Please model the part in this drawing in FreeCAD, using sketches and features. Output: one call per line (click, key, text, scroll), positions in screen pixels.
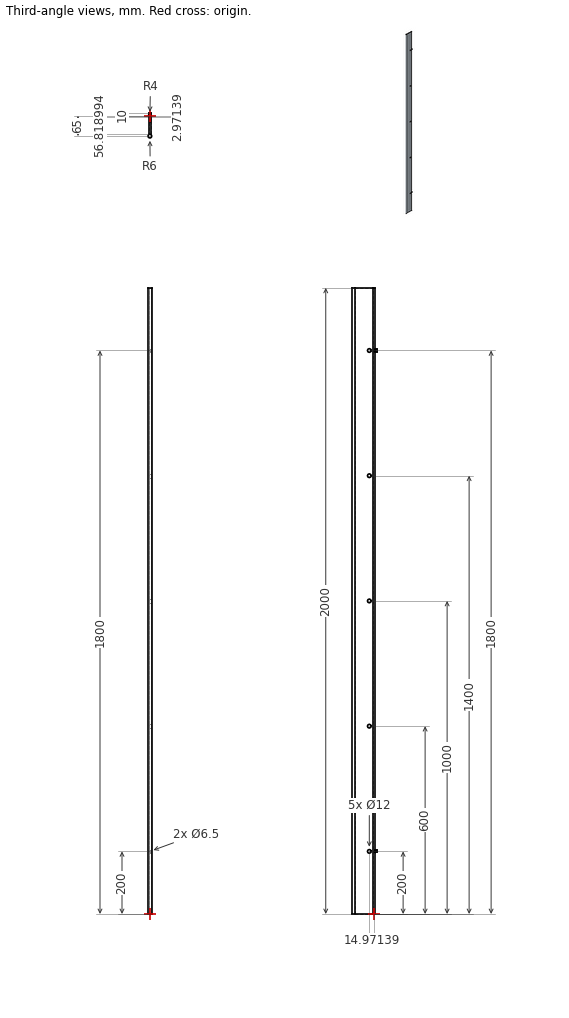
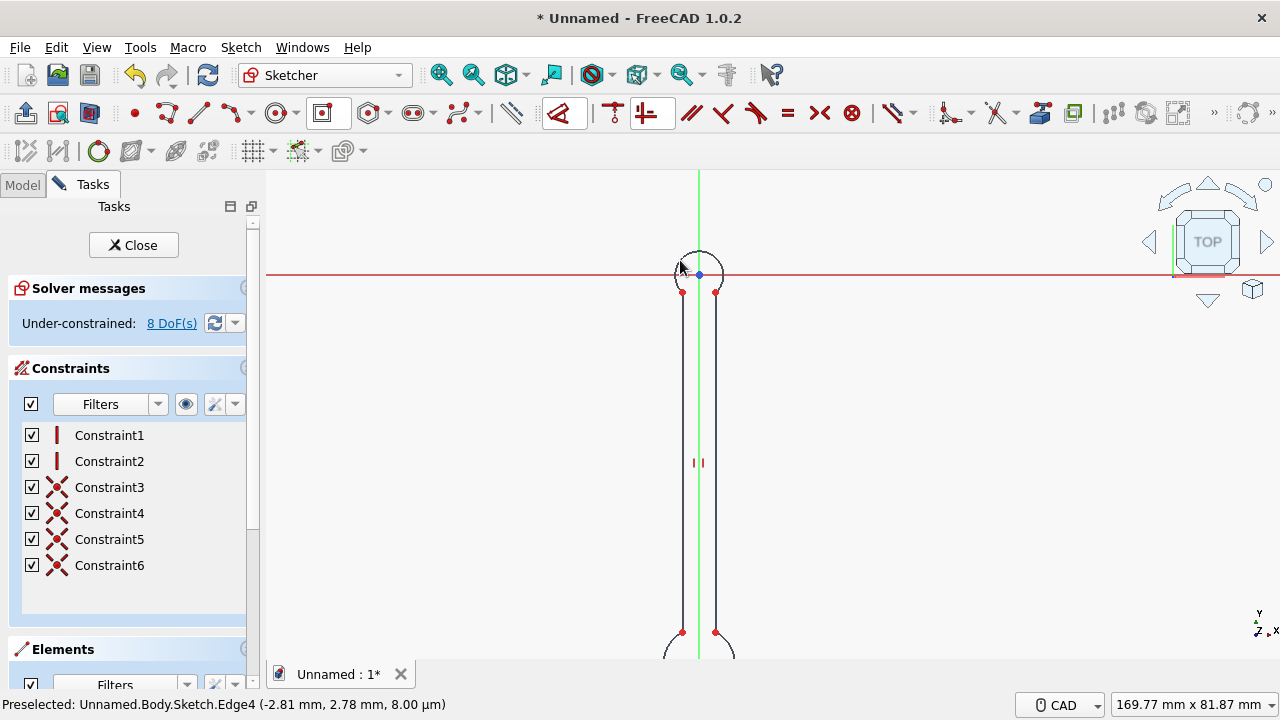
scroll(699, 275, up, 3)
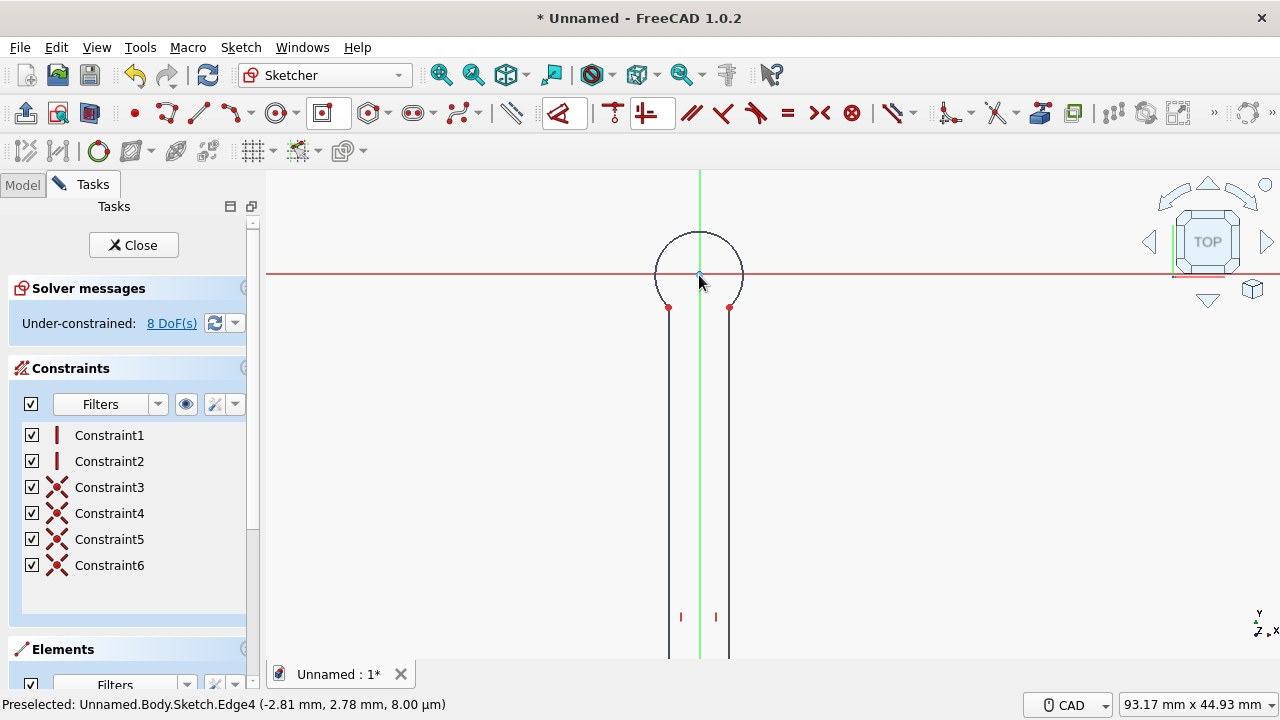
drag(689, 264, 710, 286)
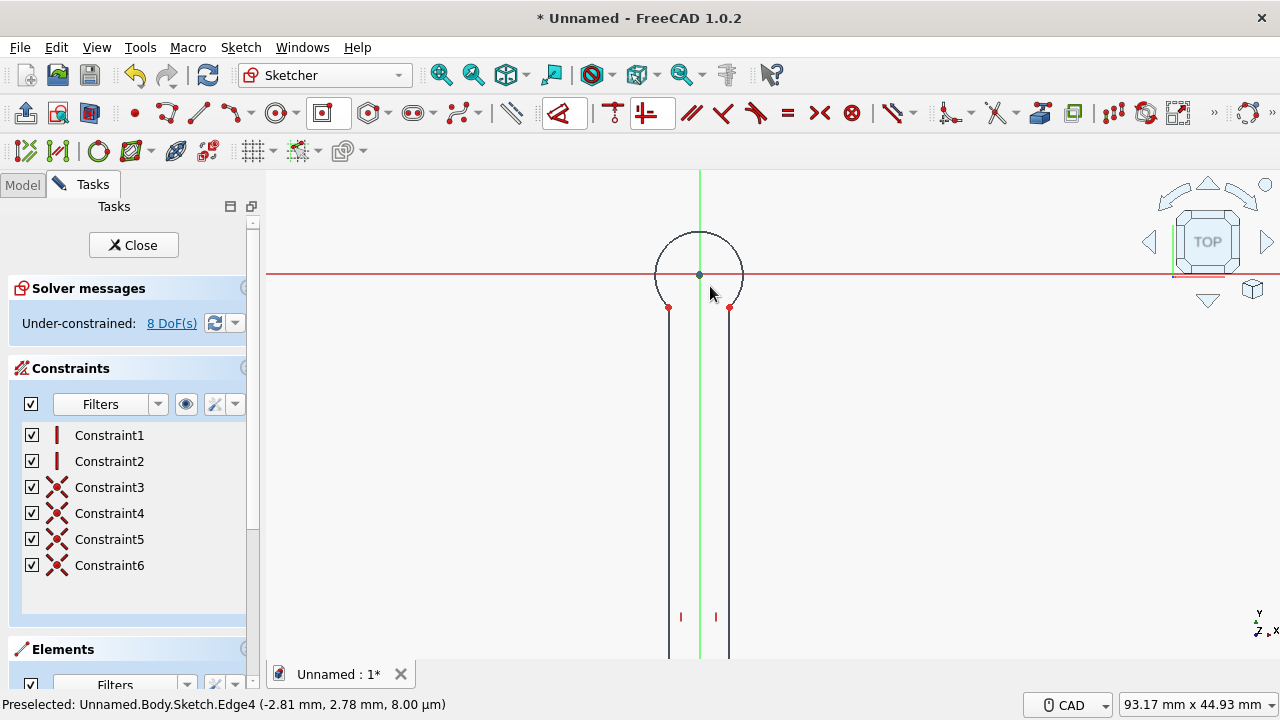
key(c)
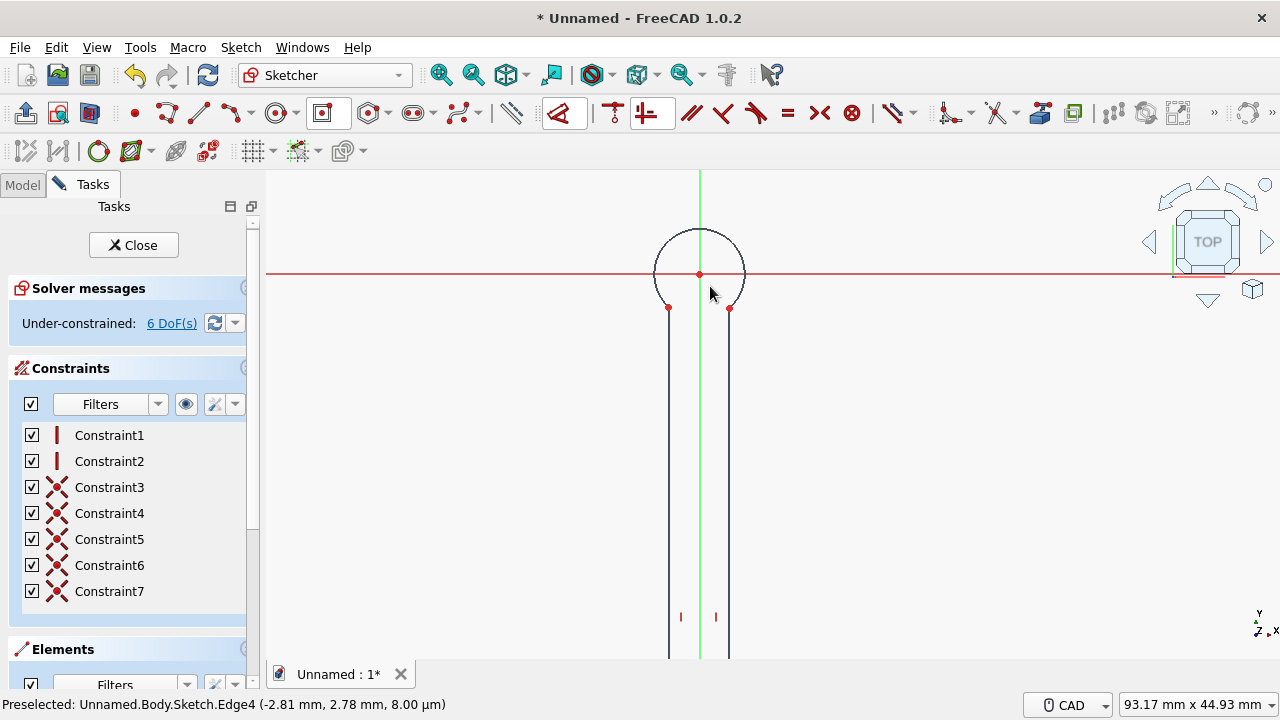
scroll(708, 284, down, 5)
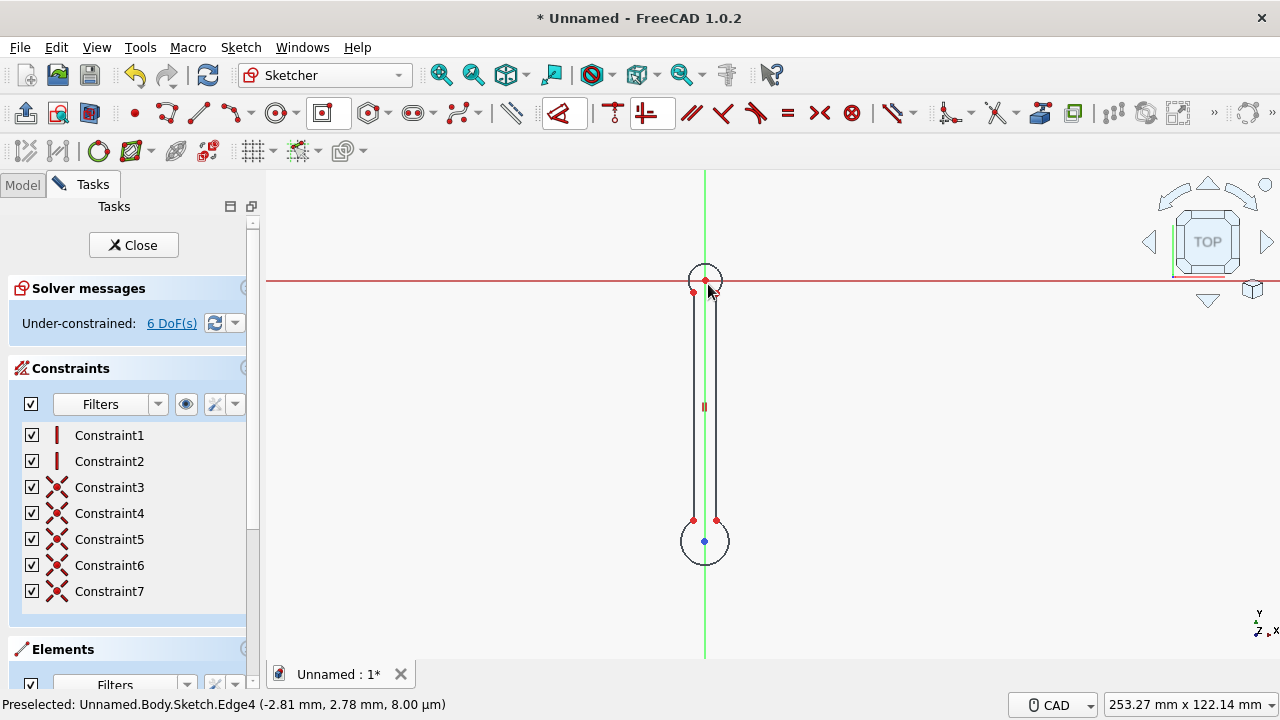
click(705, 541)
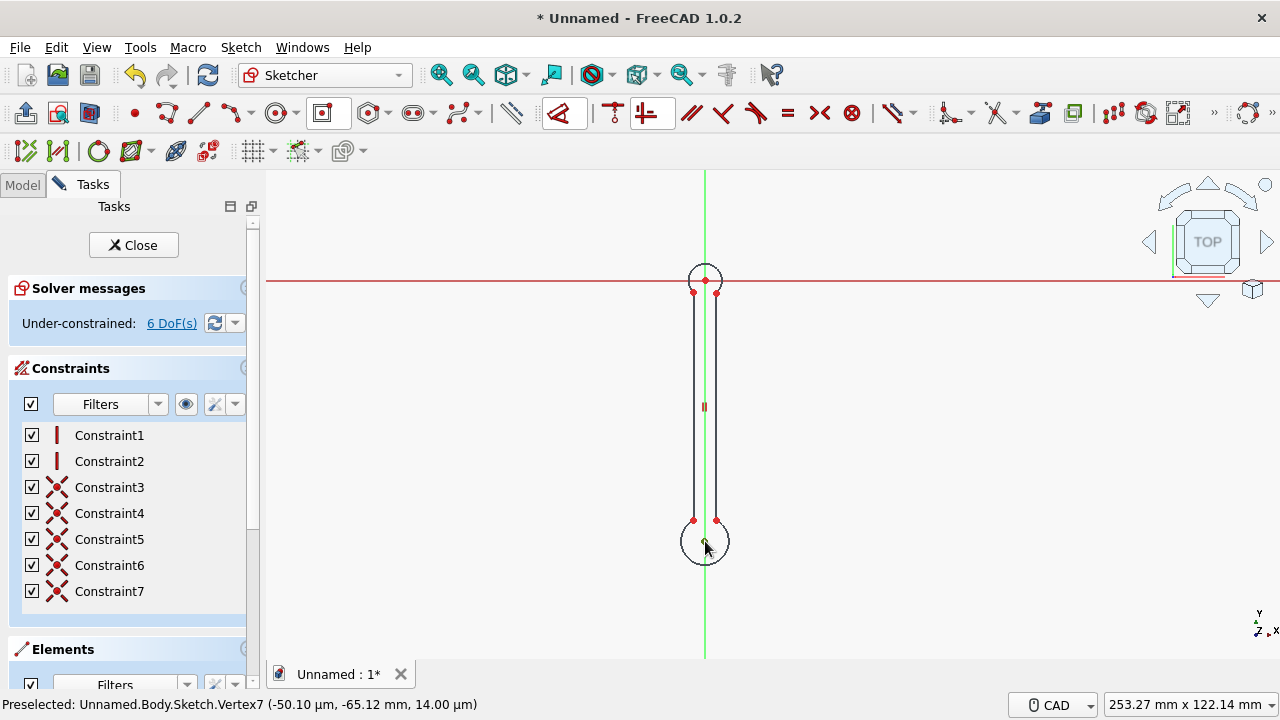
click(705, 600)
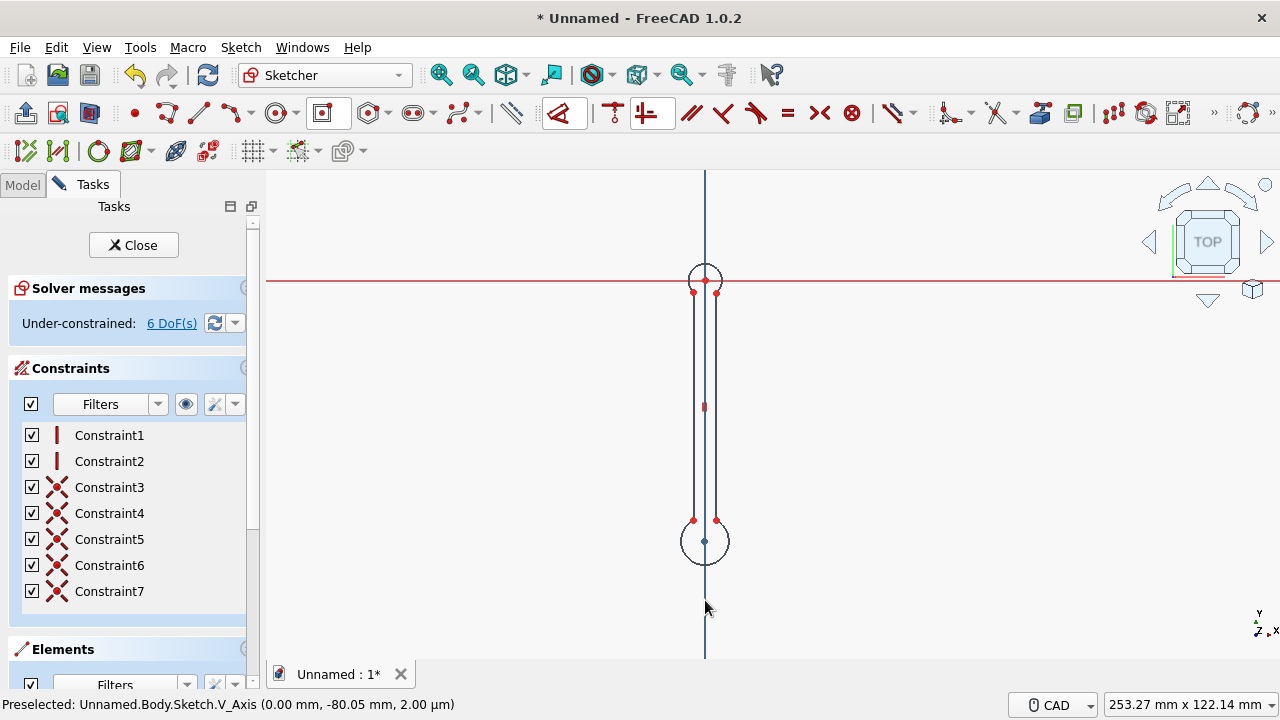
click(614, 114)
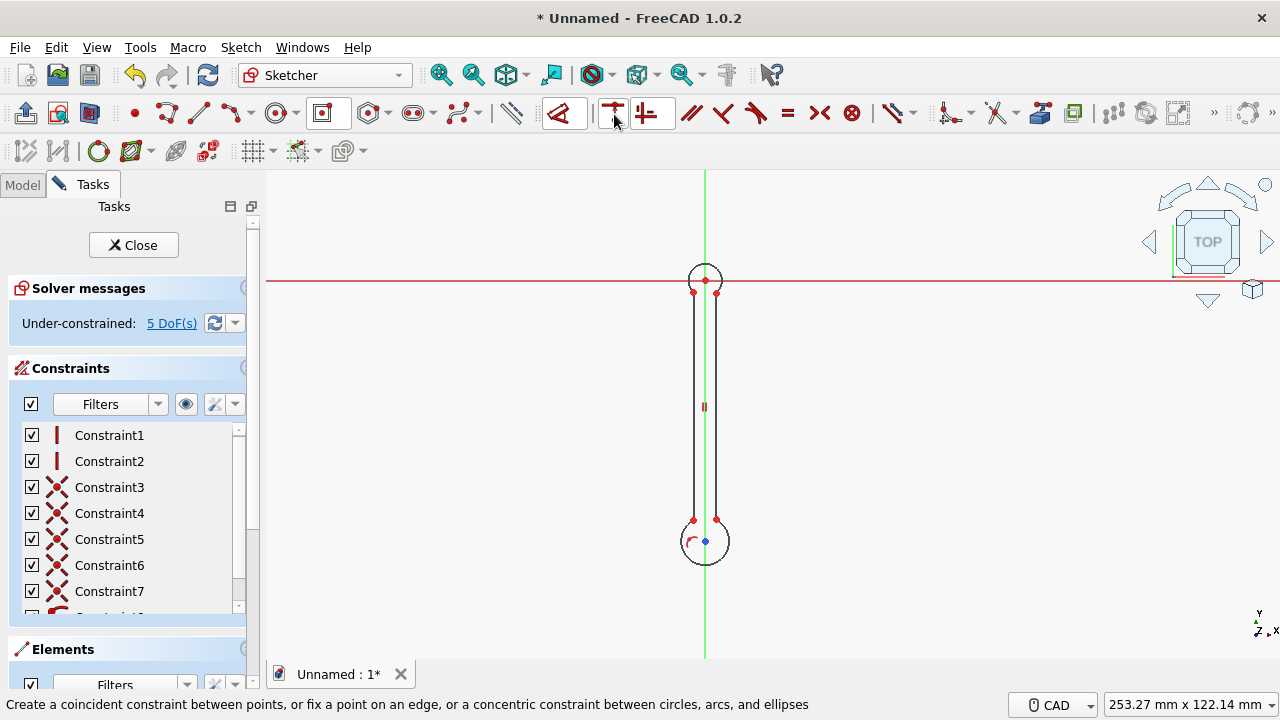
click(558, 114)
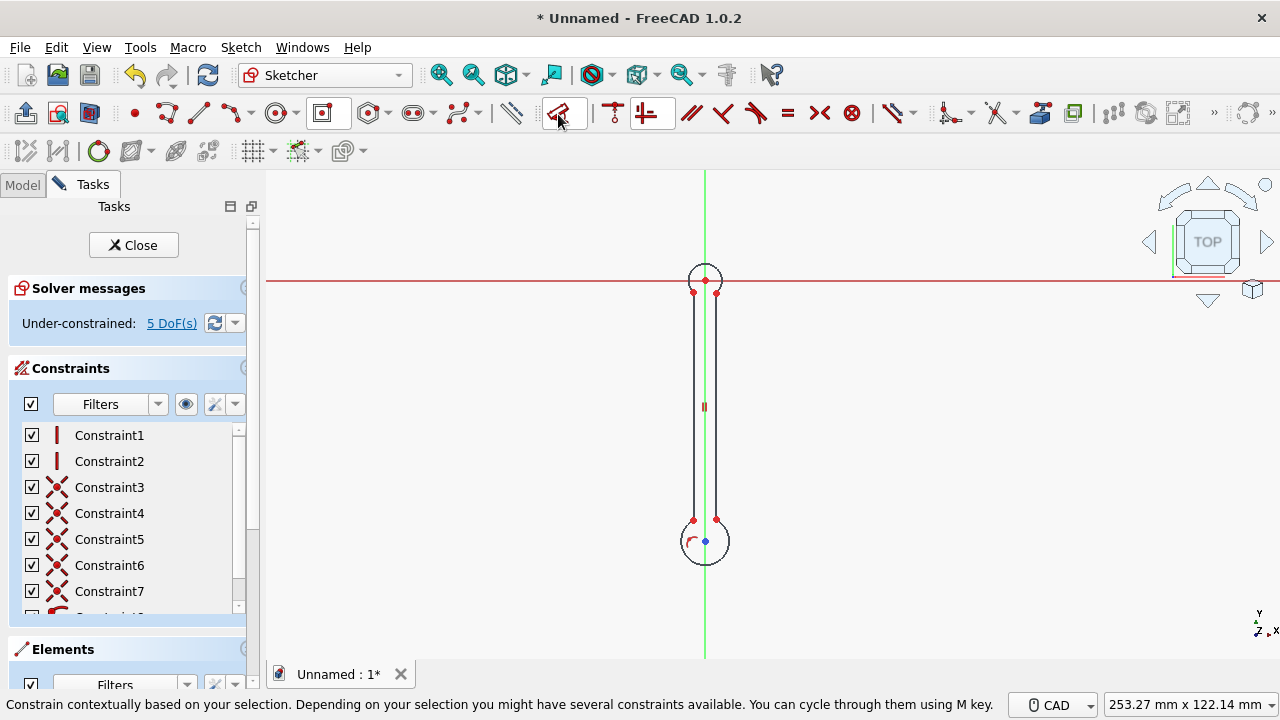
scroll(684, 553, up, 3)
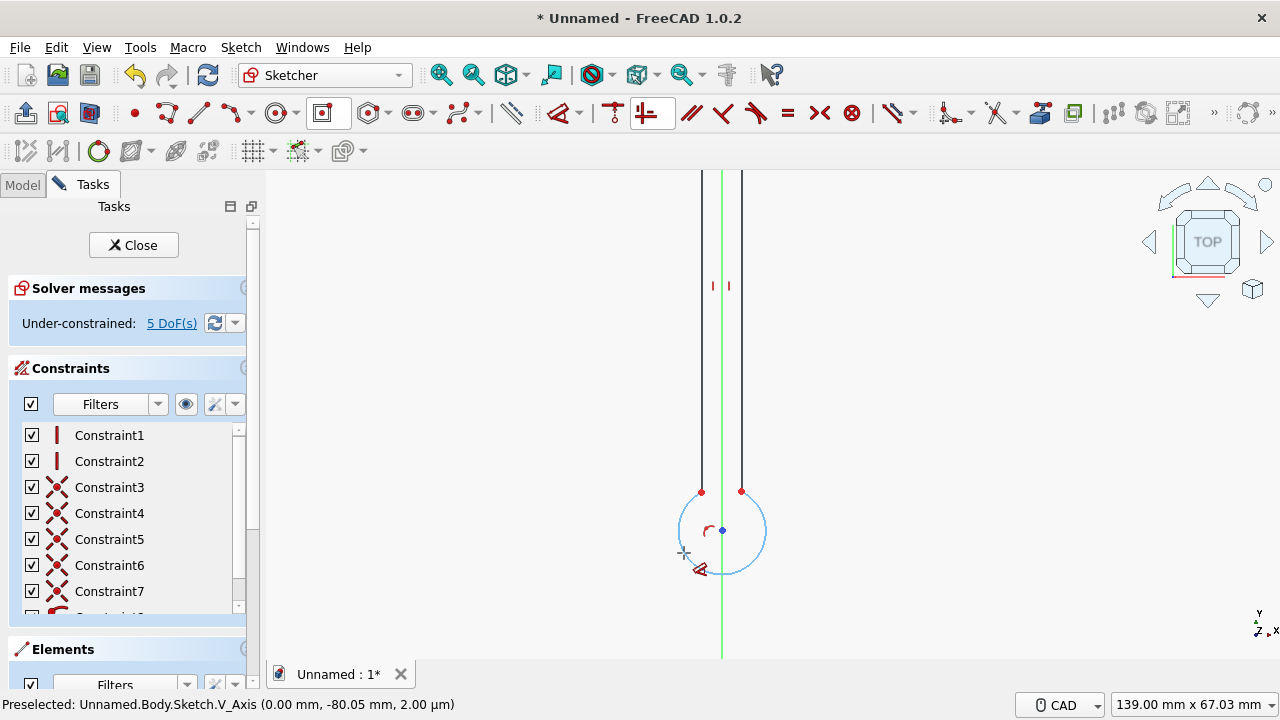
click(684, 552)
click(656, 567)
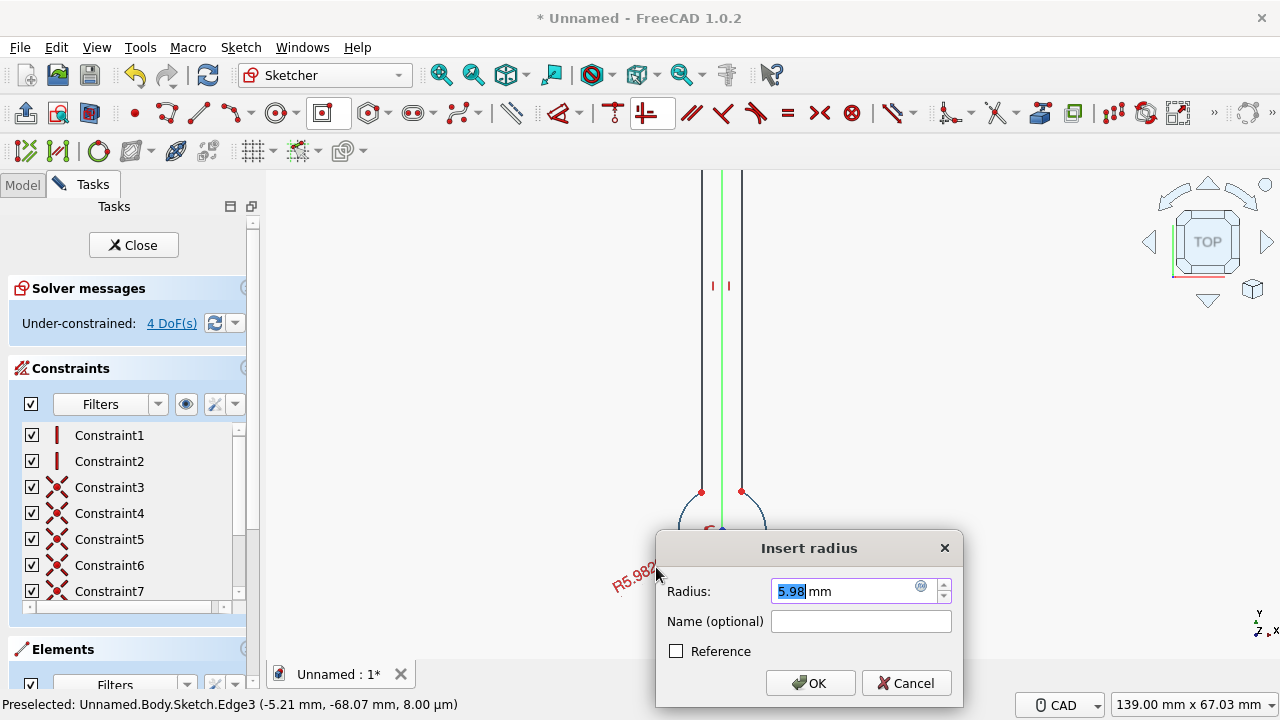
text(6)
key(Return)